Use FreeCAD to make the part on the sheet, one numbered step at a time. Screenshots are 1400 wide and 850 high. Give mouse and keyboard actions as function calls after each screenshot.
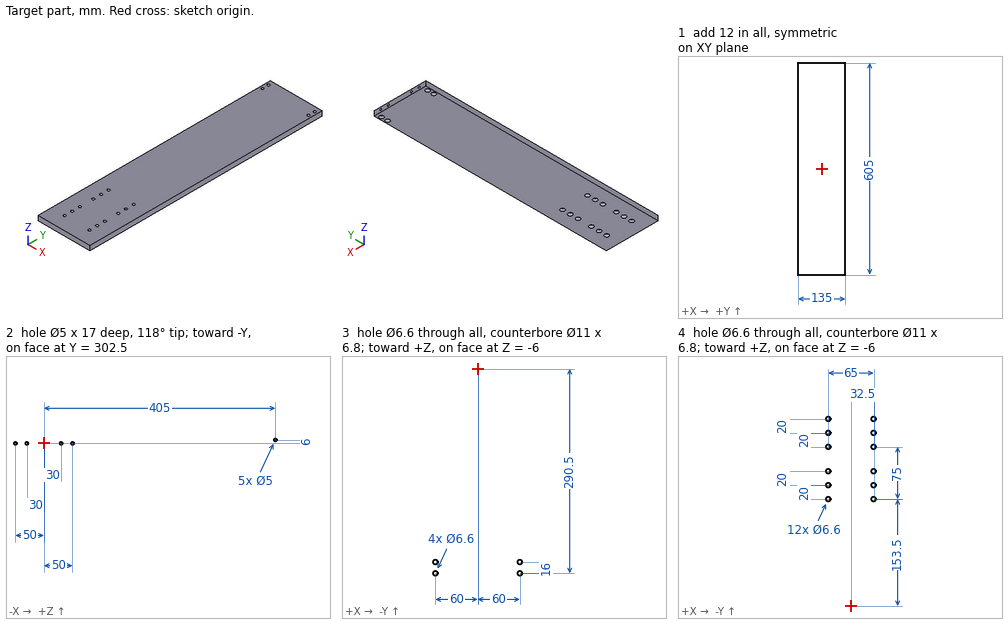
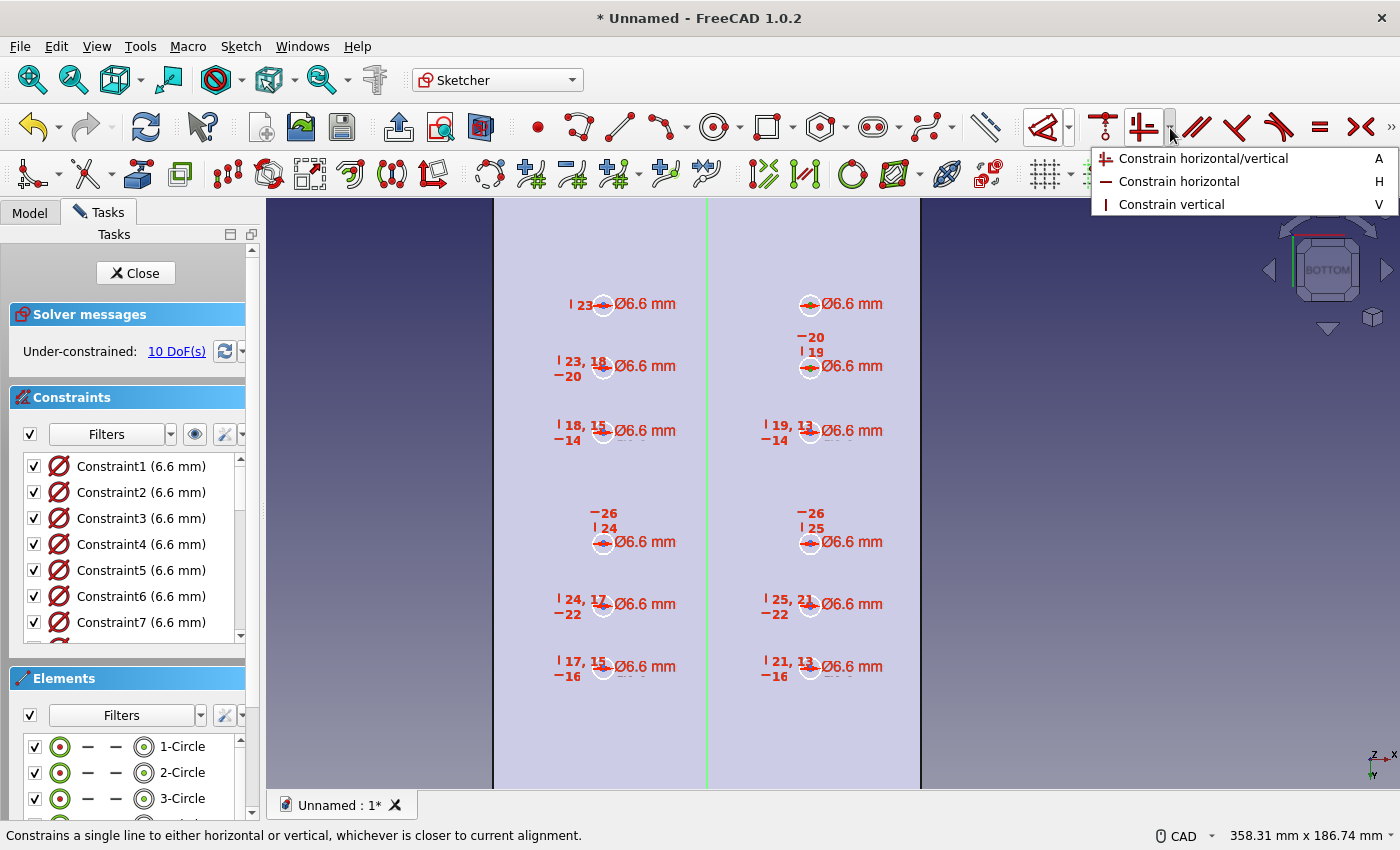
click(1245, 204)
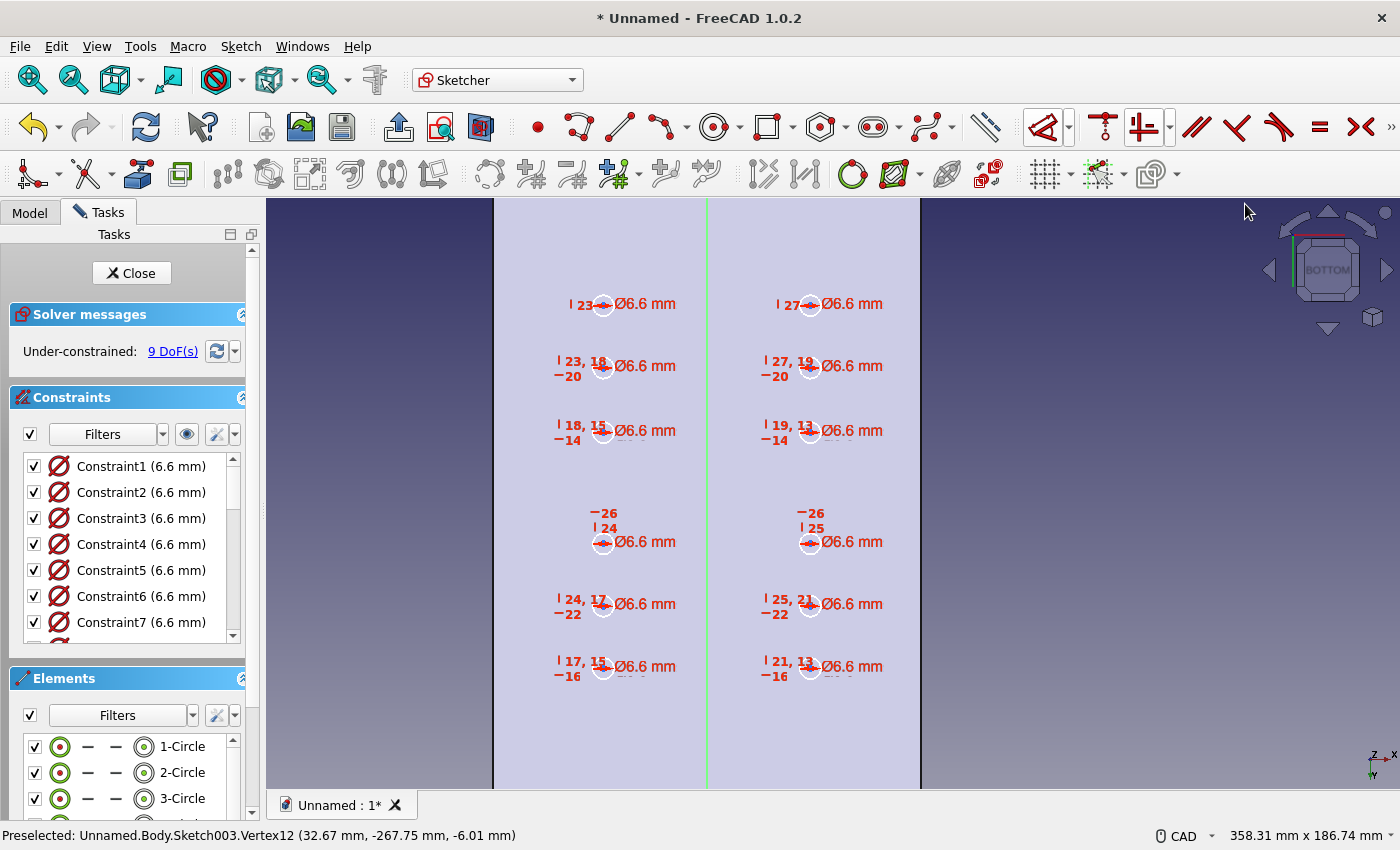
click(603, 306)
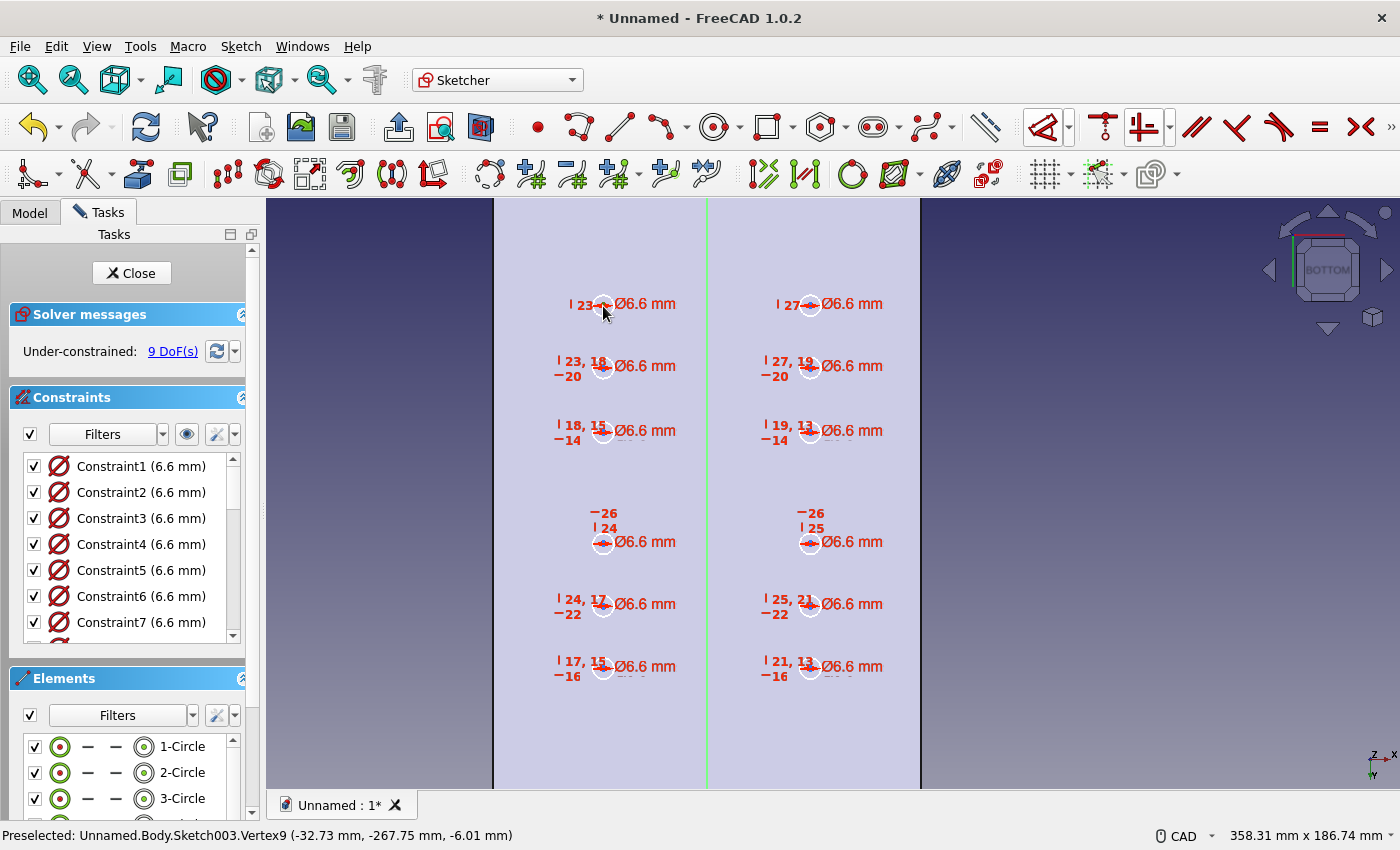
click(810, 306)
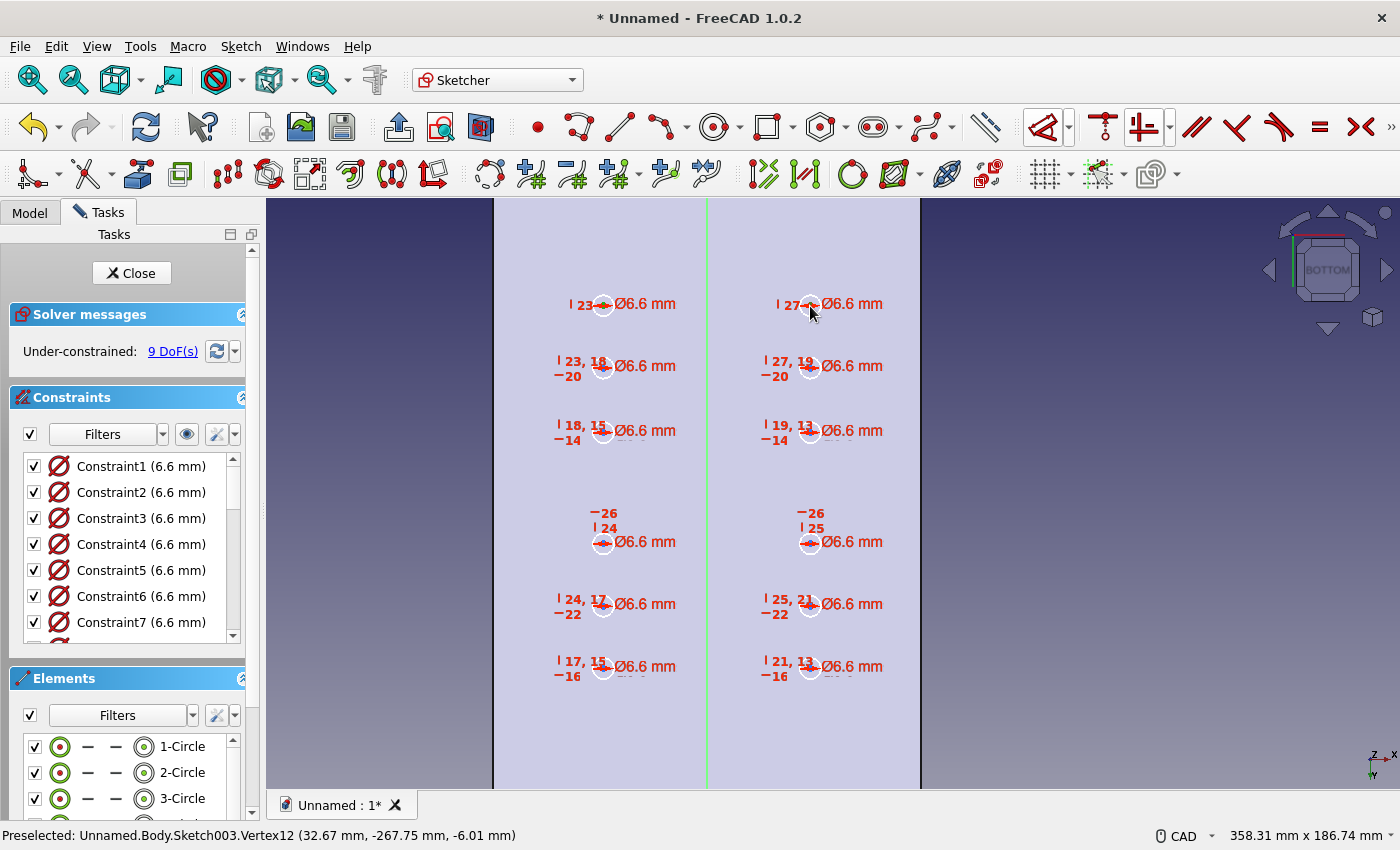
click(1170, 128)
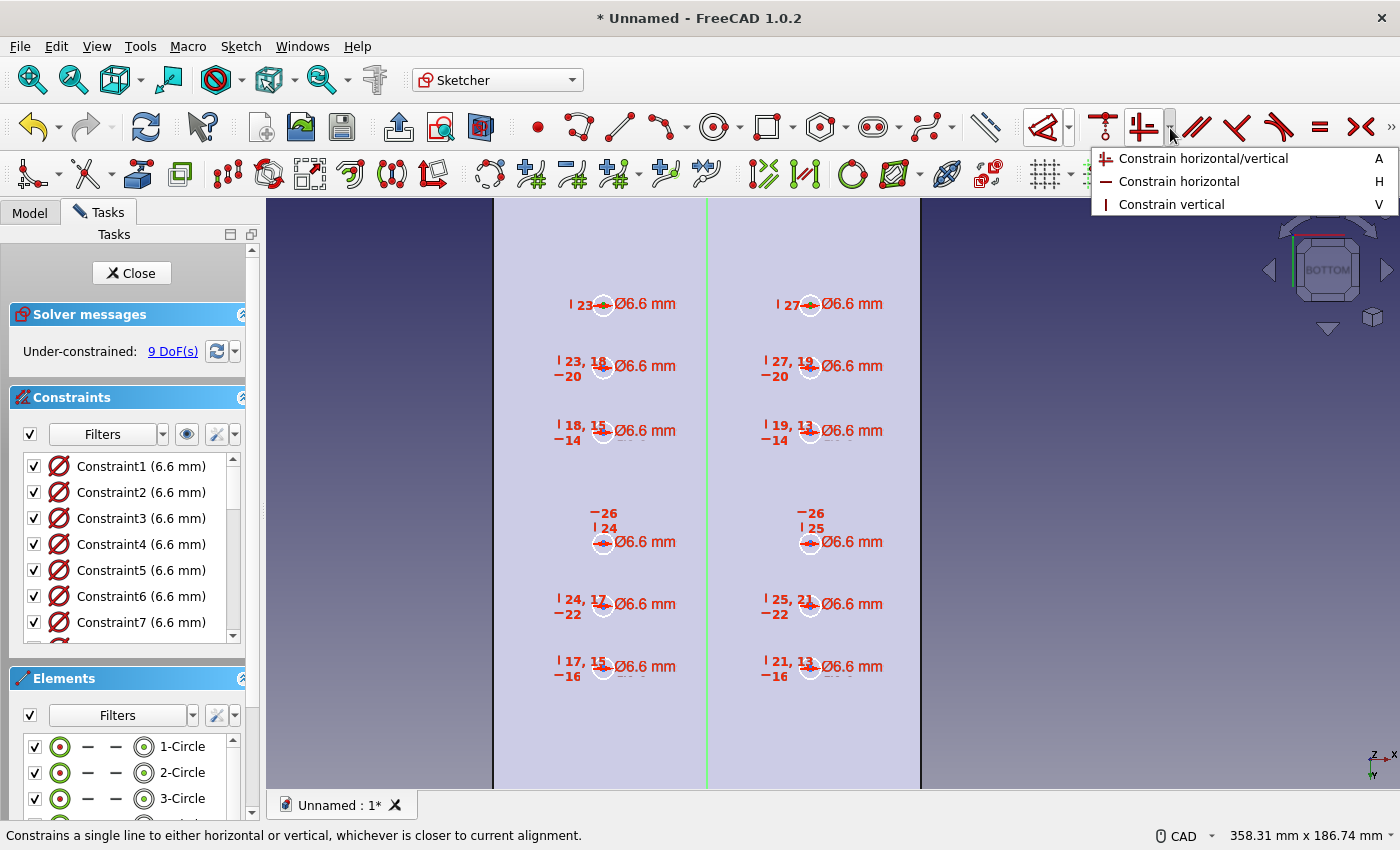
click(1245, 182)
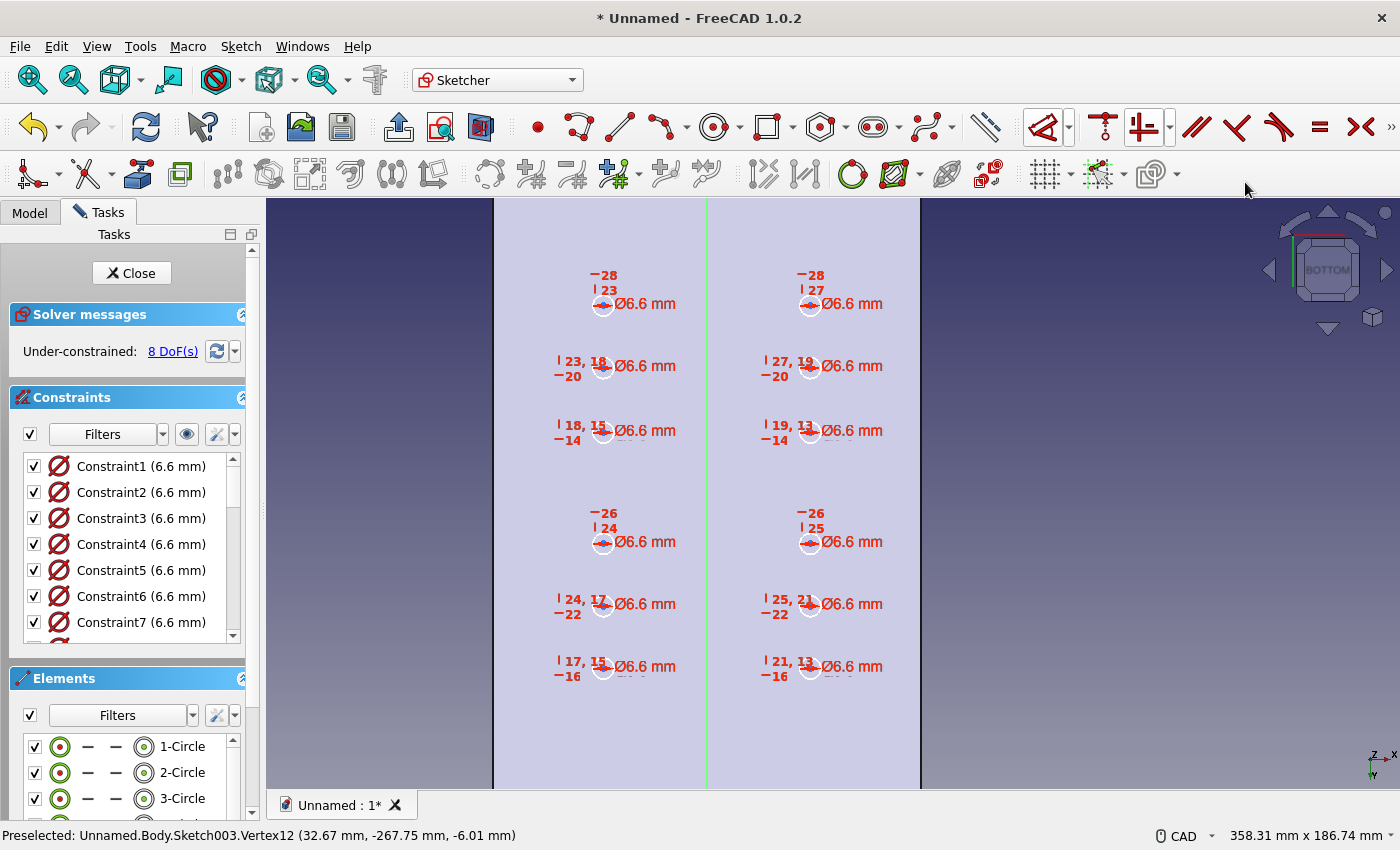
click(810, 669)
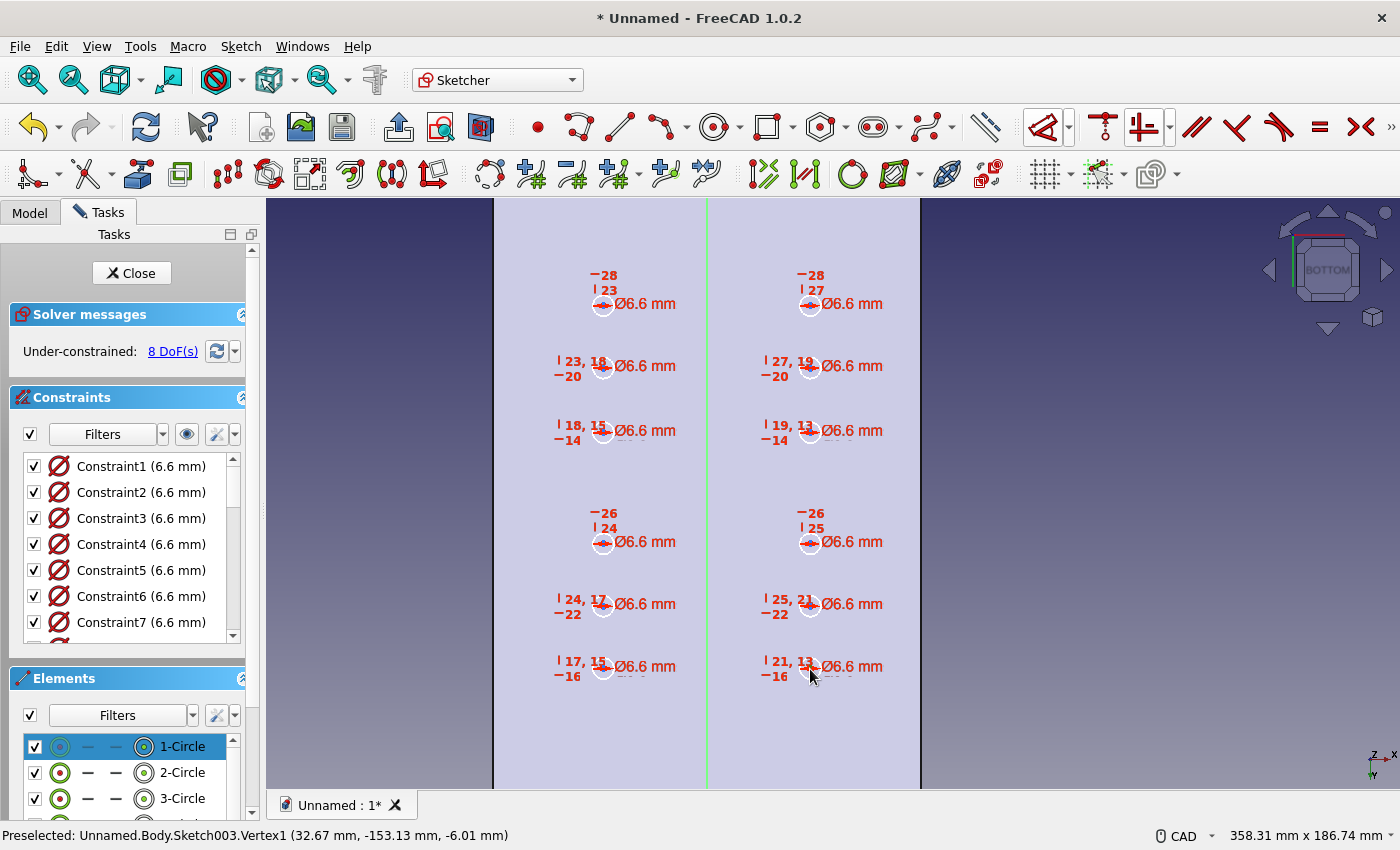
click(810, 433)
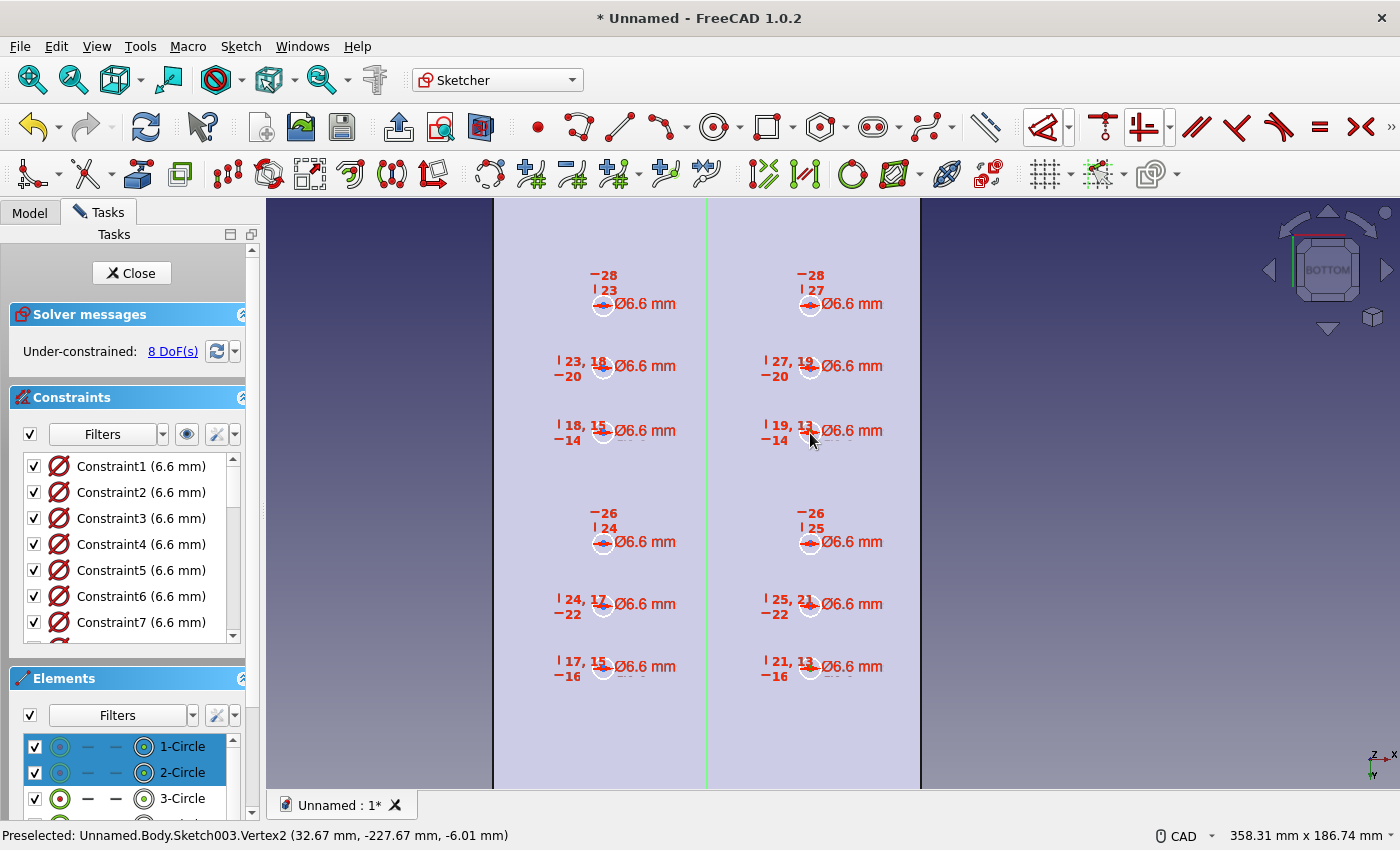
key(i)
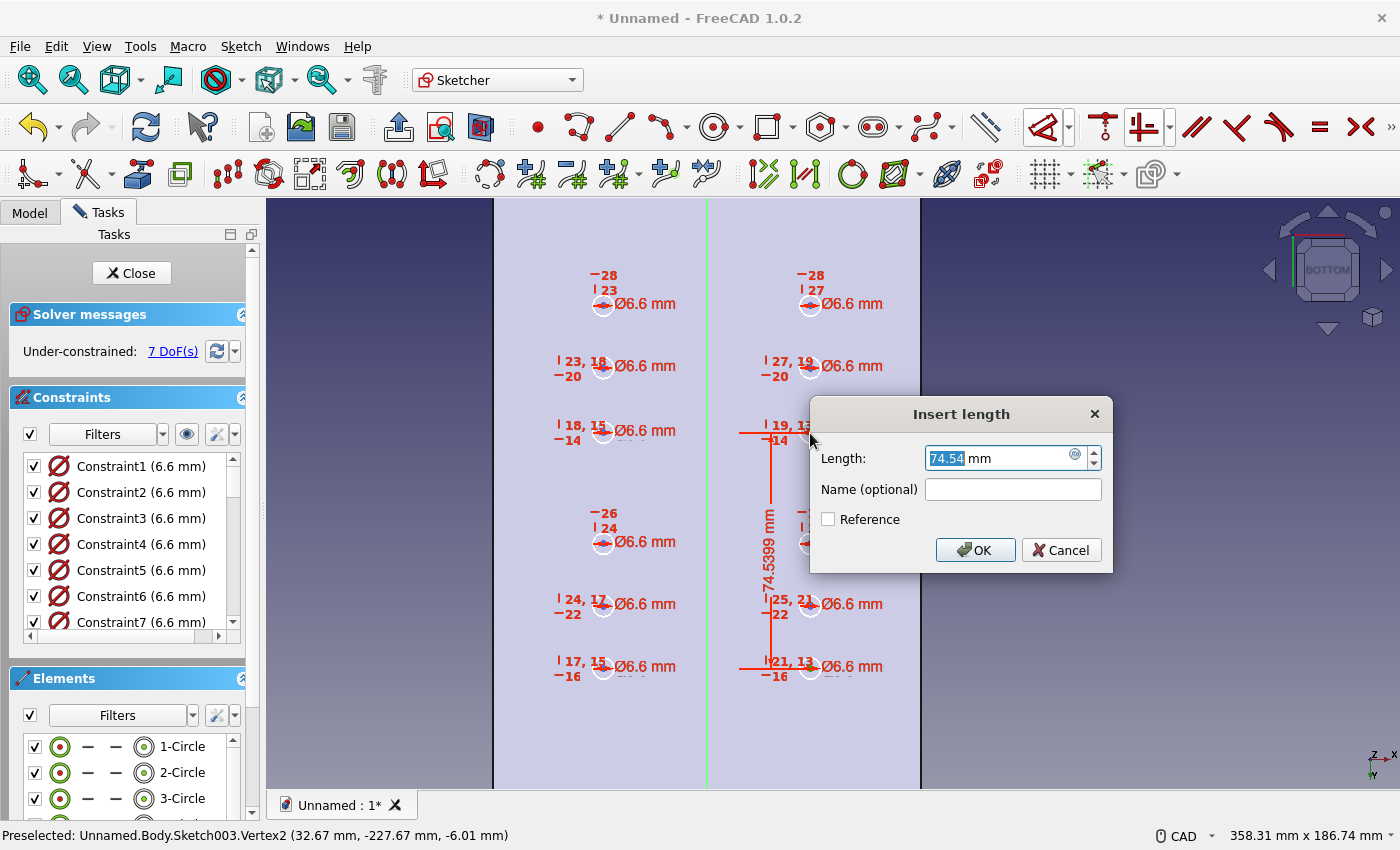
text(75)
key(Return)